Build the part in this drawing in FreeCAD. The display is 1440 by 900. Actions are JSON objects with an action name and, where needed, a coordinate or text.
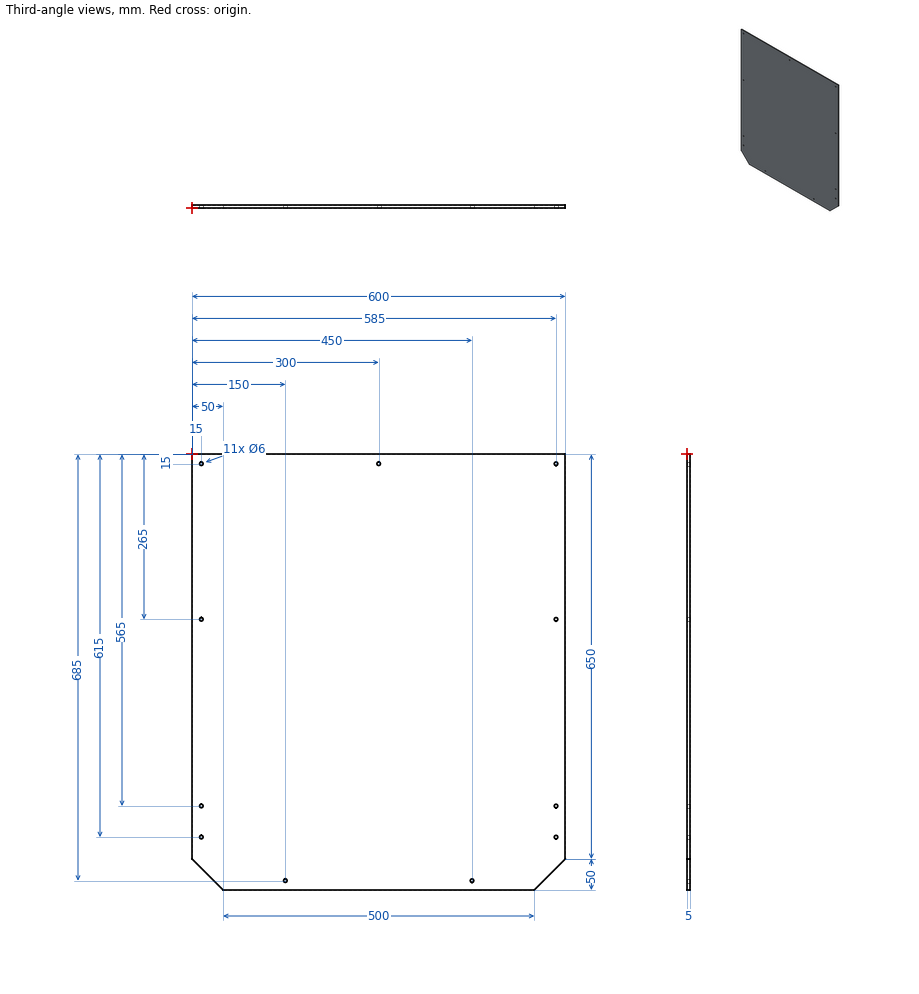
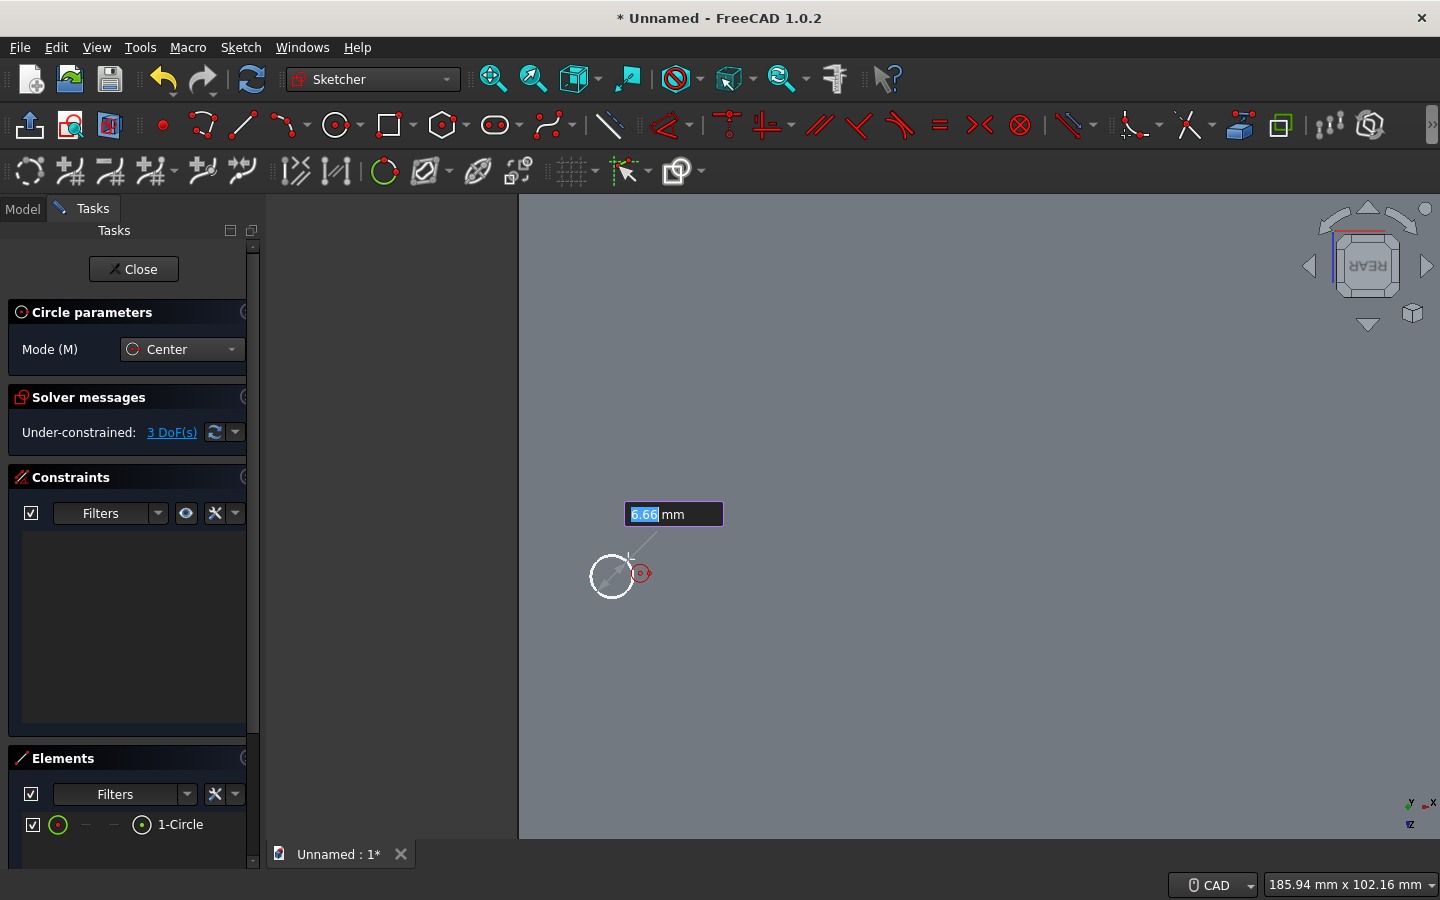
{"action": "left_click", "coordinate": [626, 559]}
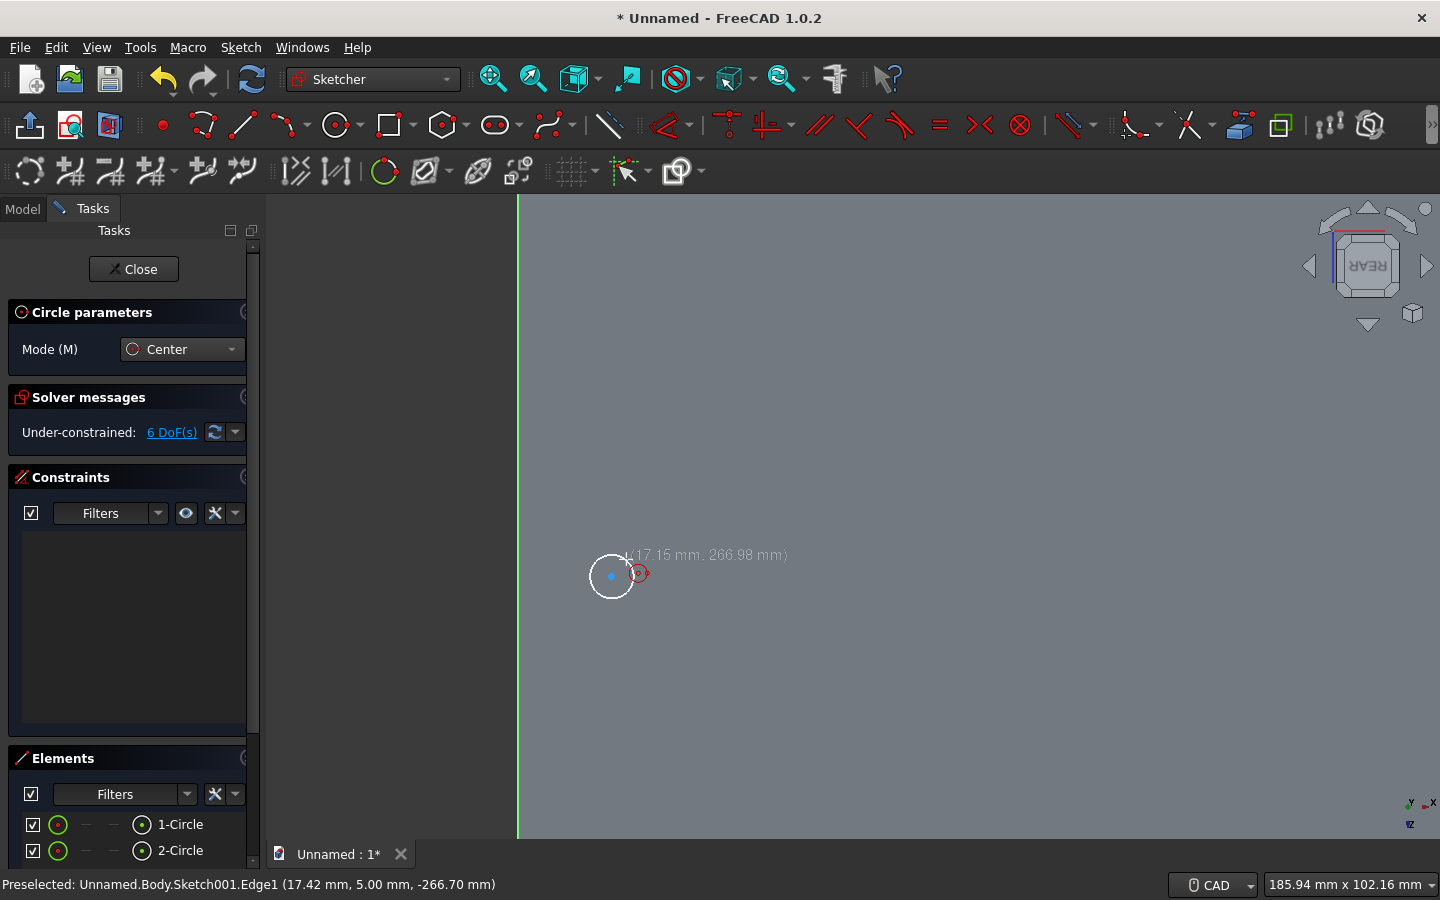
{"action": "scroll", "coordinate": [626, 561], "scroll_direction": "down", "scroll_amount": 12}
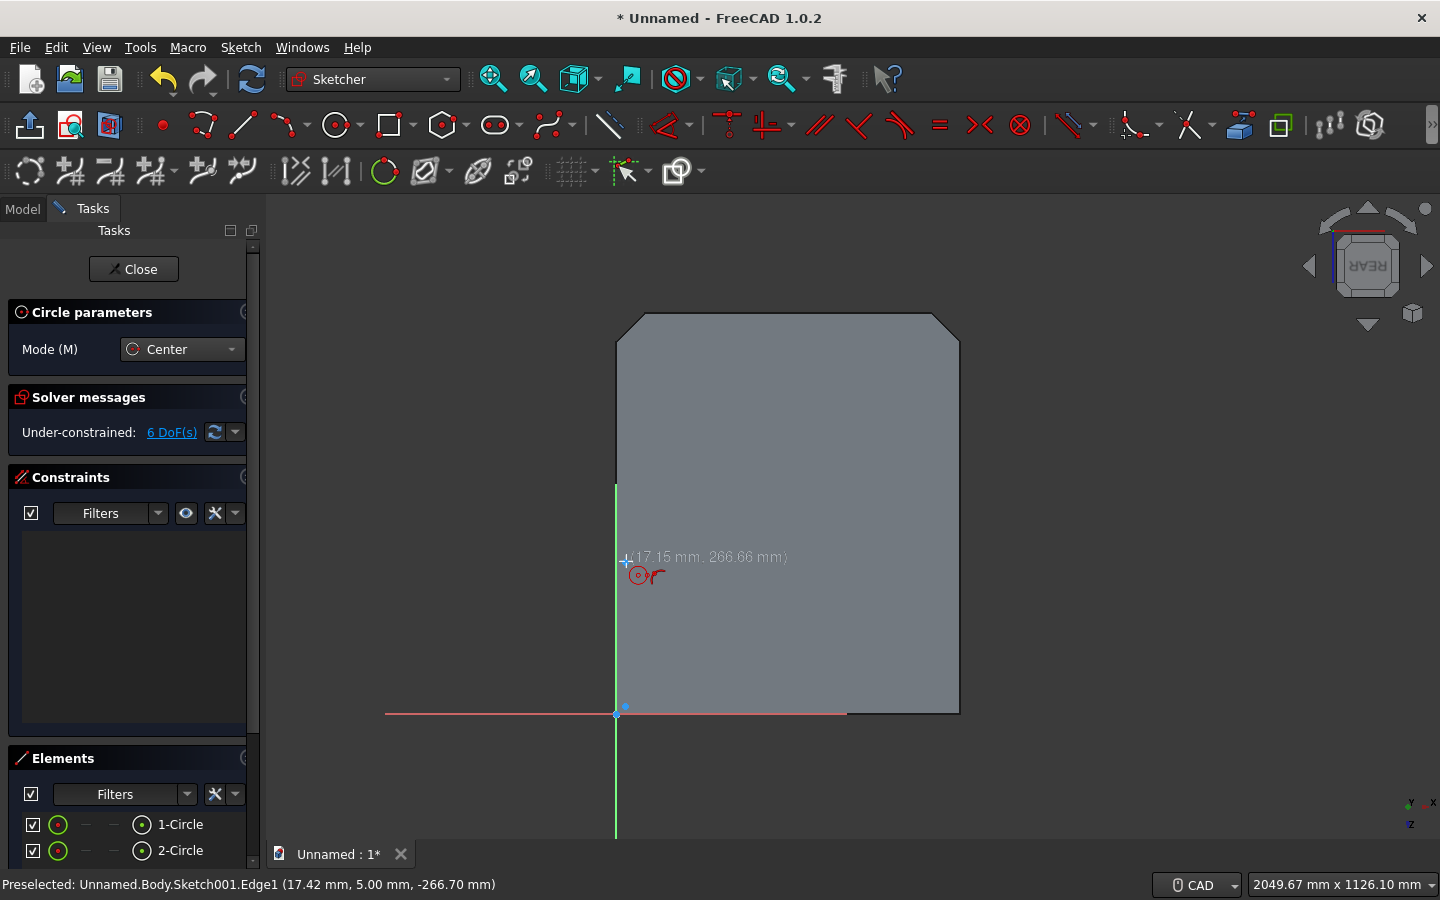
{"action": "scroll", "coordinate": [625, 391], "scroll_direction": "up", "scroll_amount": 13}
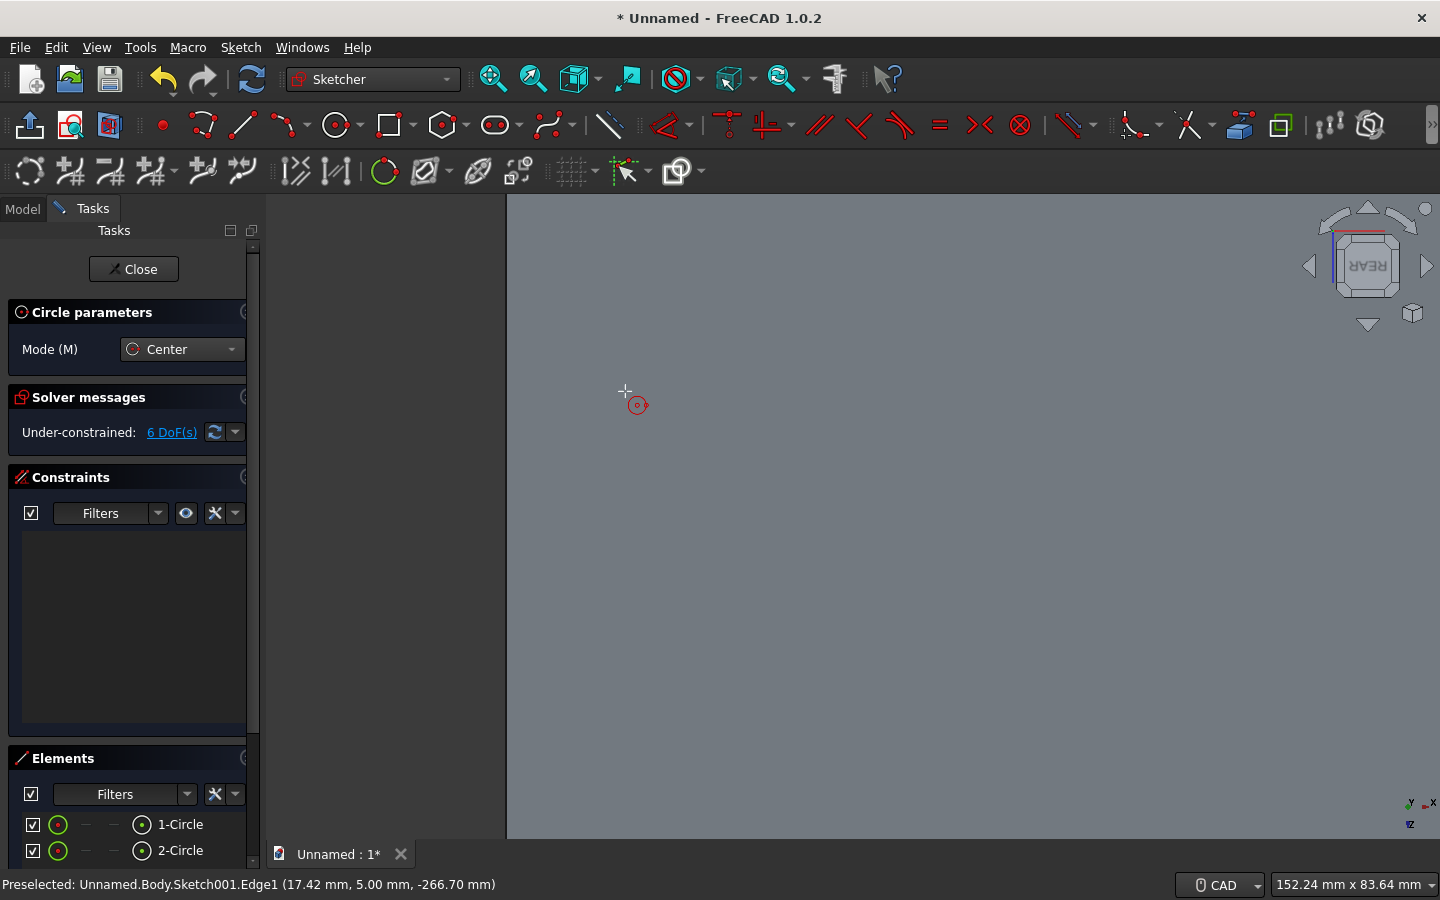
{"action": "scroll", "coordinate": [625, 390], "scroll_direction": "down", "scroll_amount": 13}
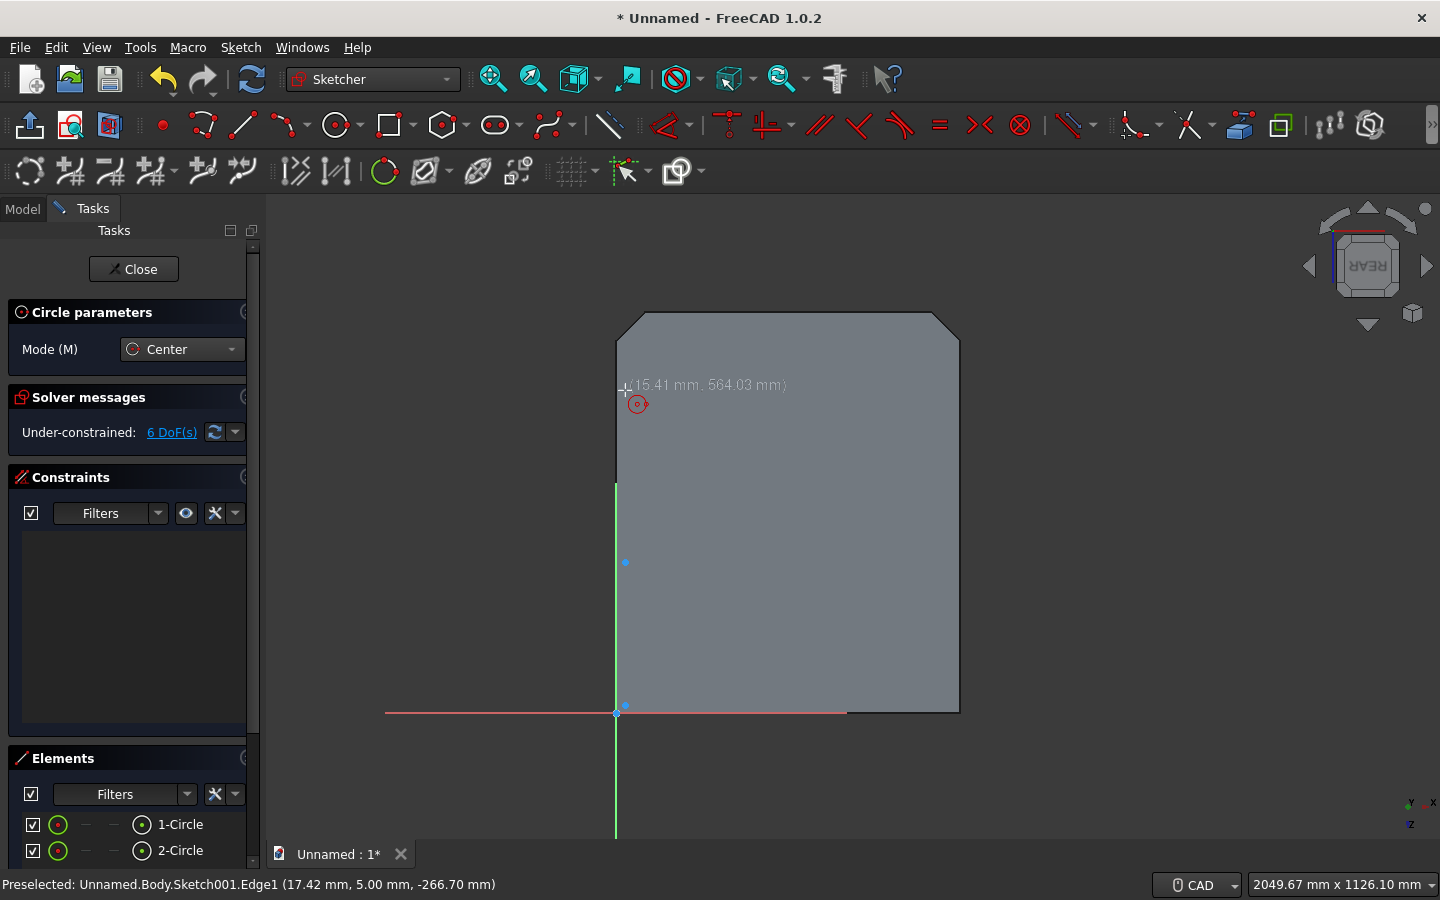
{"action": "scroll", "coordinate": [625, 390], "scroll_direction": "up", "scroll_amount": 4}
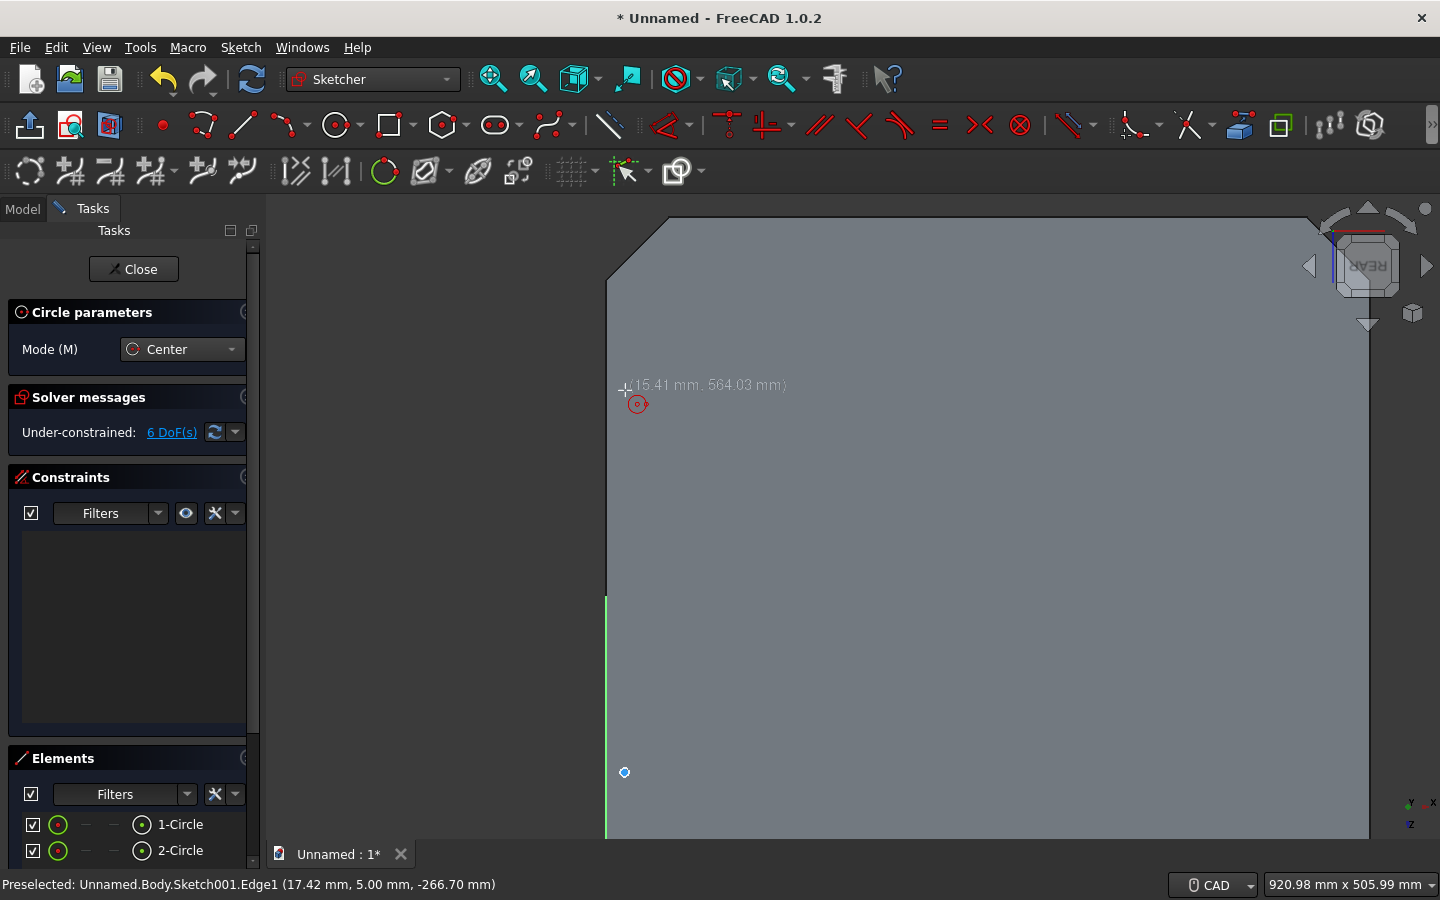
{"action": "left_click", "coordinate": [625, 389]}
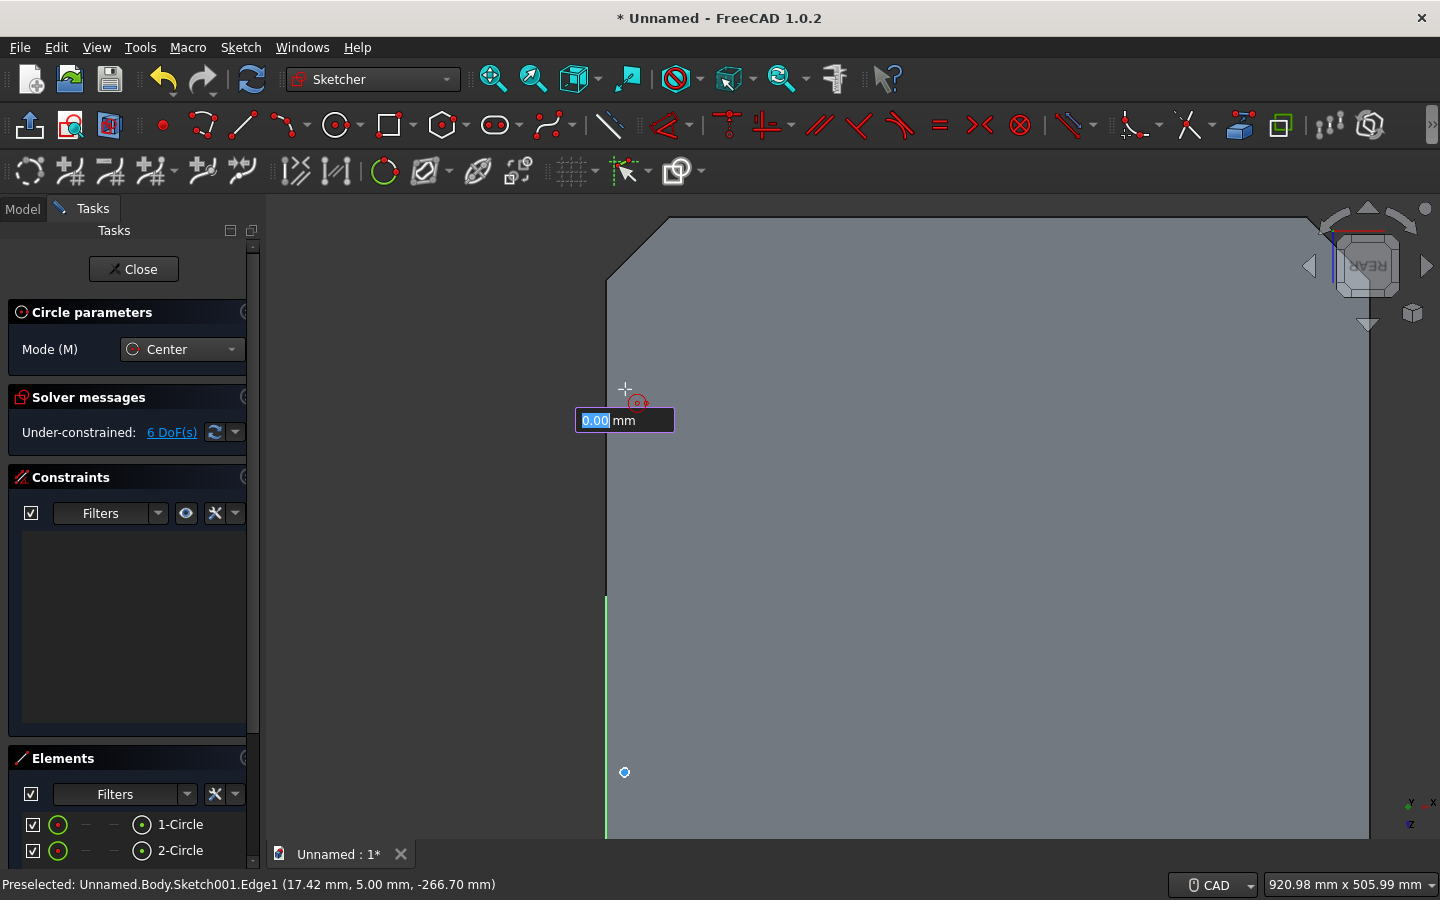
{"action": "scroll", "coordinate": [627, 386], "scroll_direction": "up", "scroll_amount": 8}